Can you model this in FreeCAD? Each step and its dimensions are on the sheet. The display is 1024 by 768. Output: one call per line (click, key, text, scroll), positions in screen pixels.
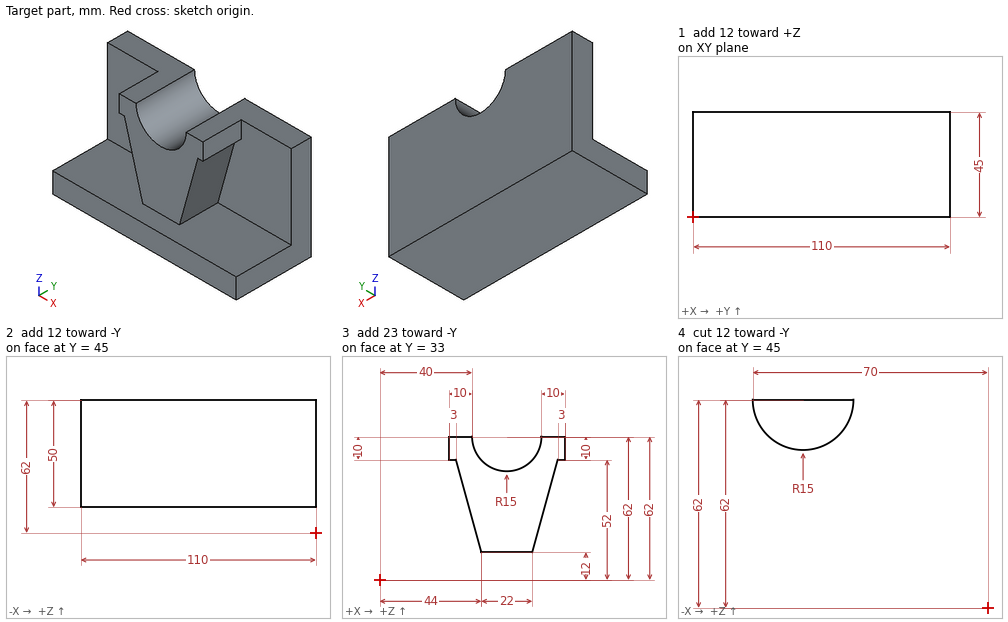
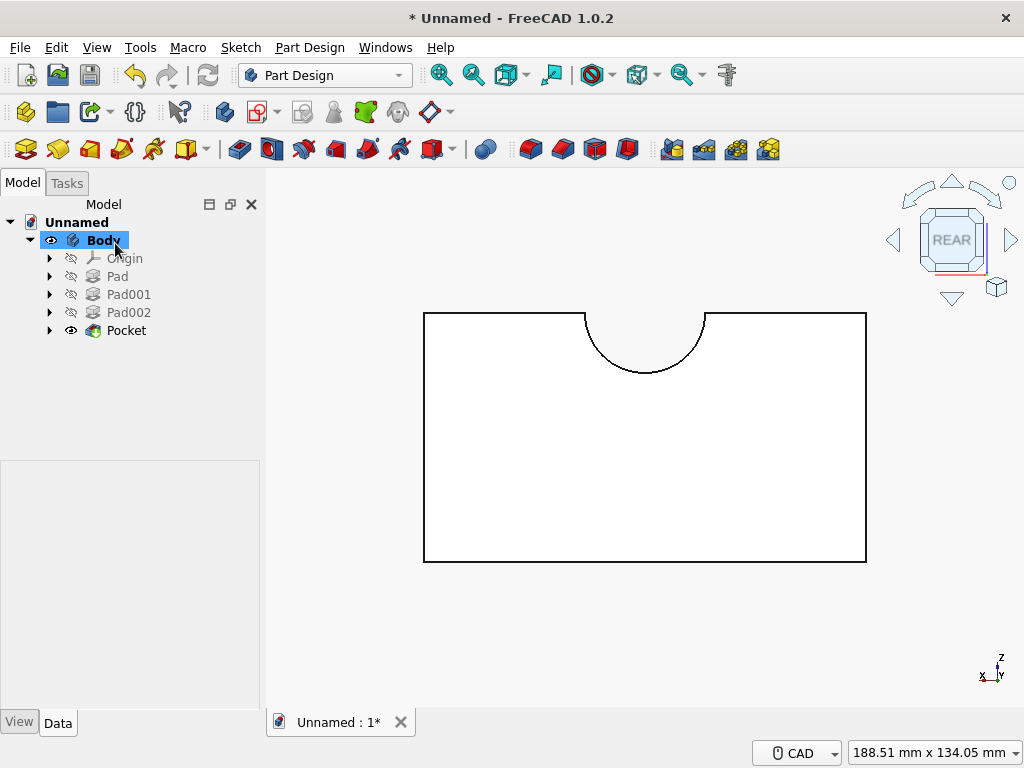
key(0)